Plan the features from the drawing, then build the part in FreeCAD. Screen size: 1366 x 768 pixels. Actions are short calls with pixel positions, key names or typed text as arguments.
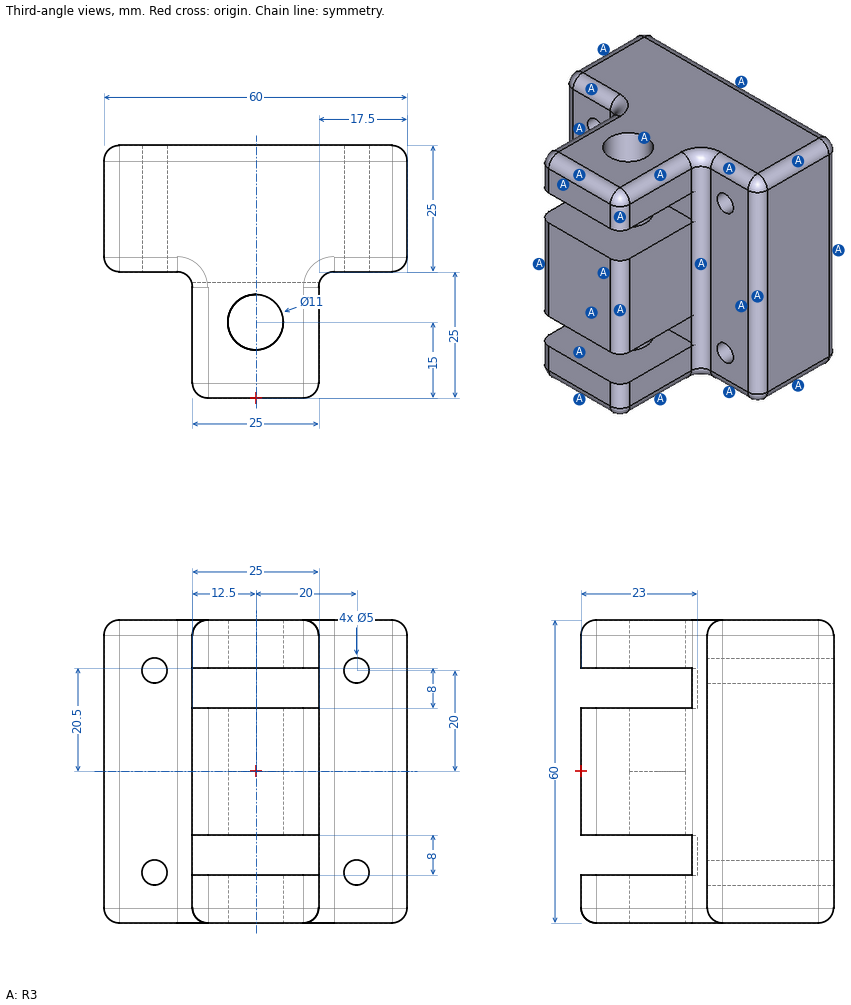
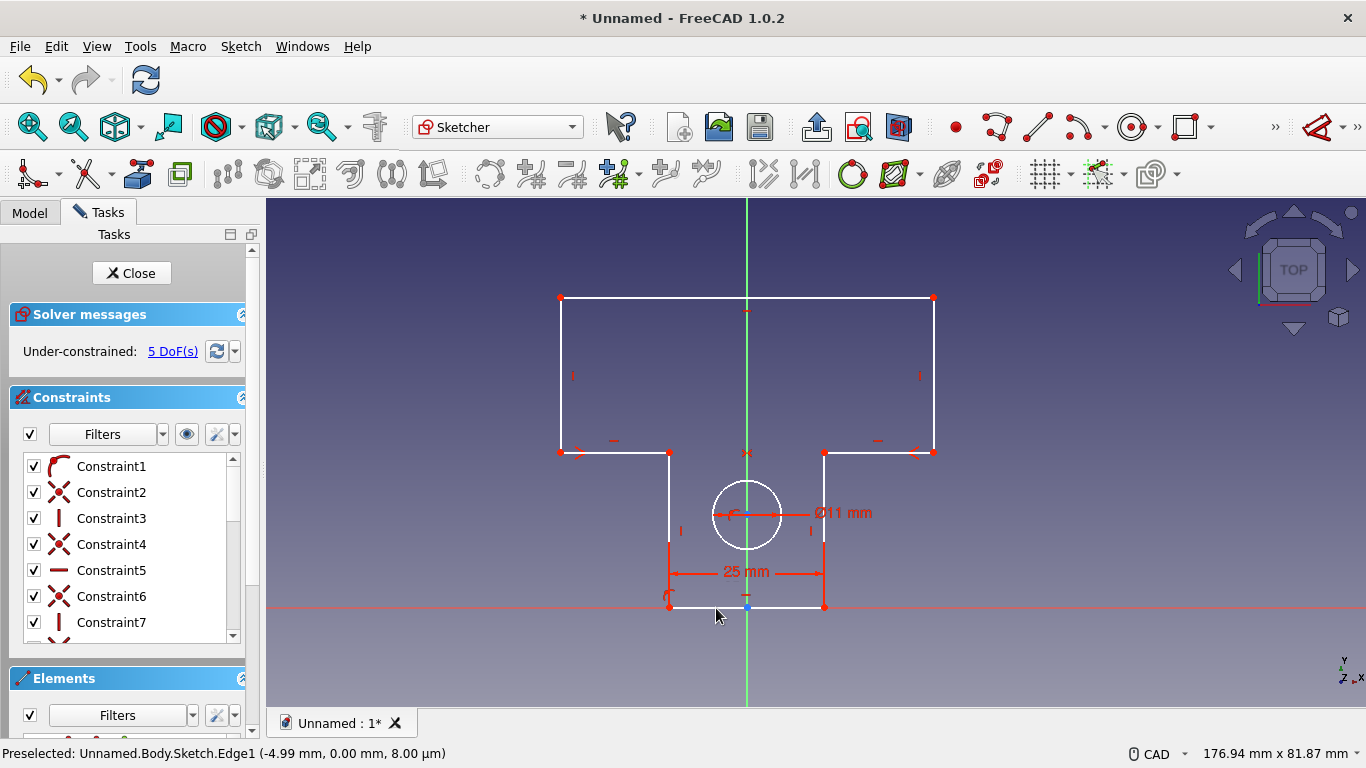
click(824, 561)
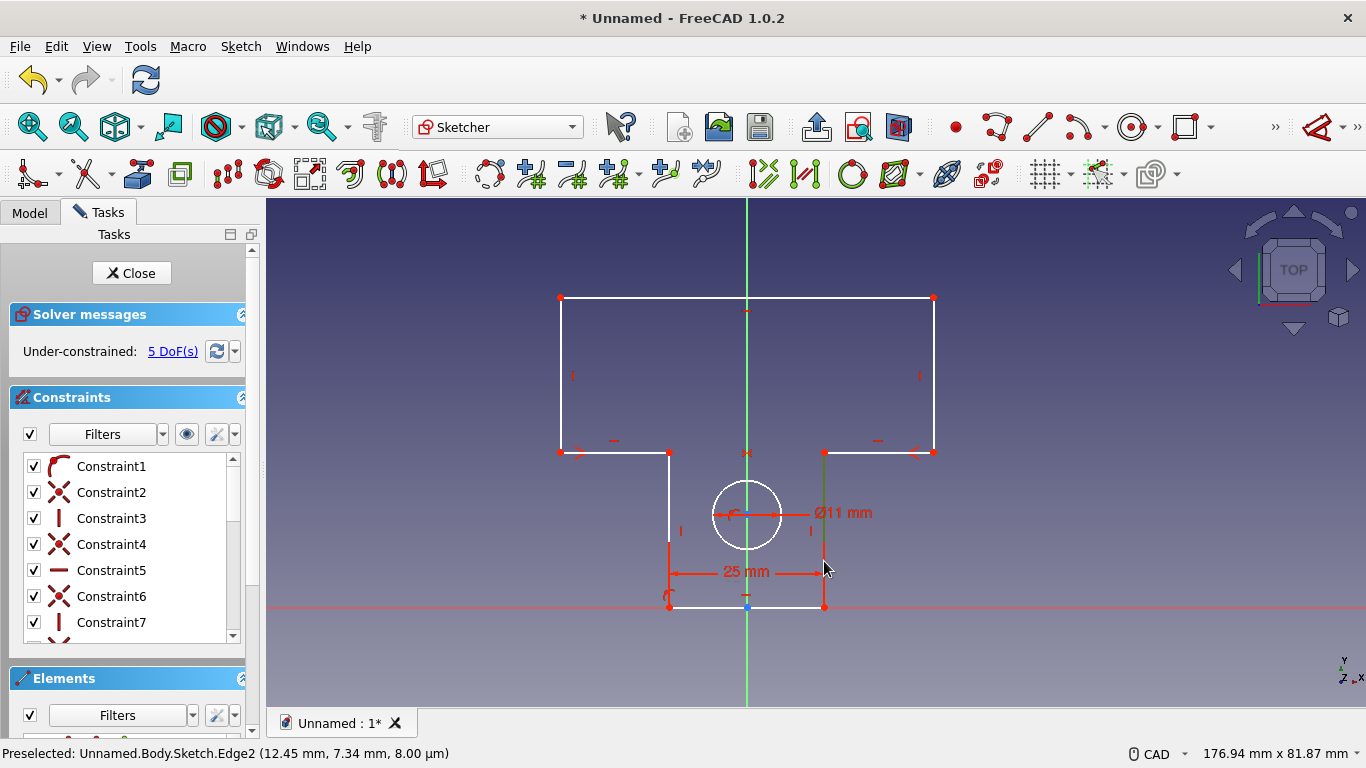
key(i)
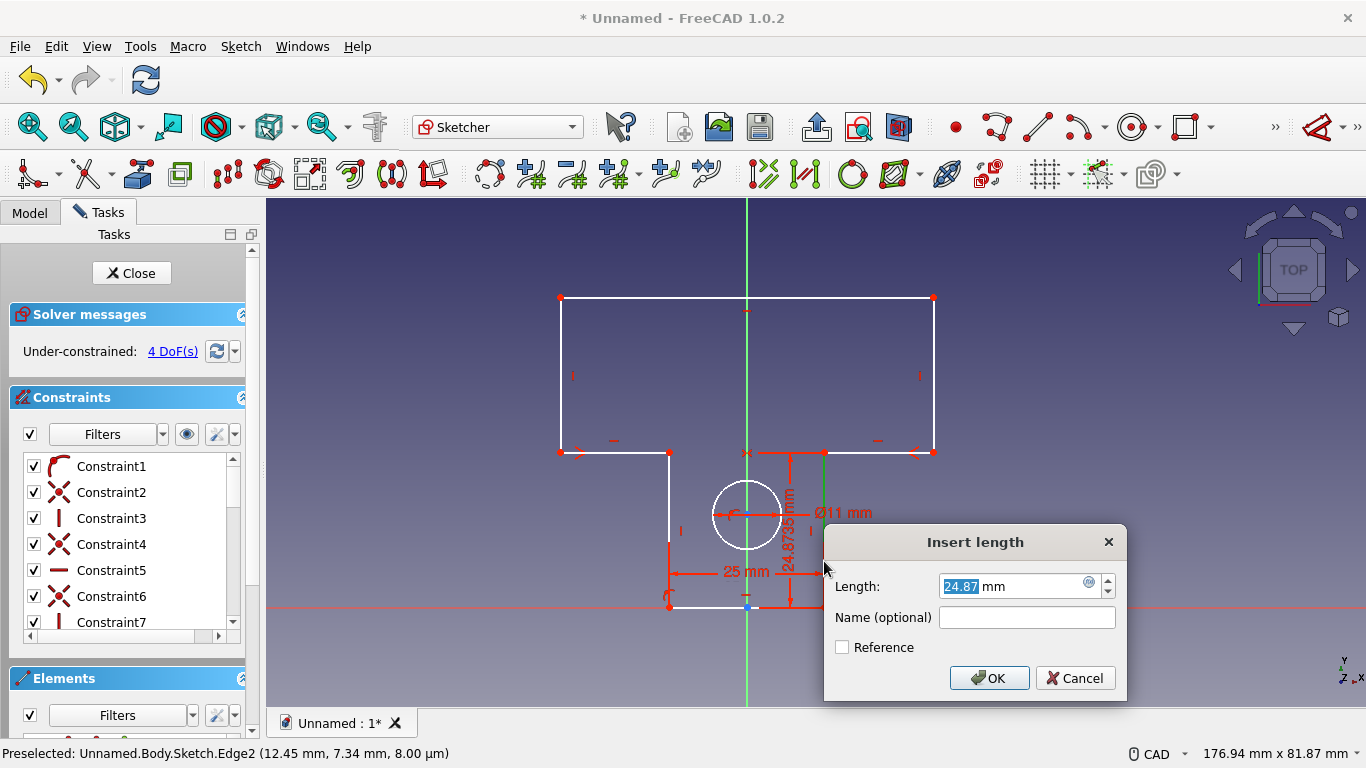
text(25)
key(Return)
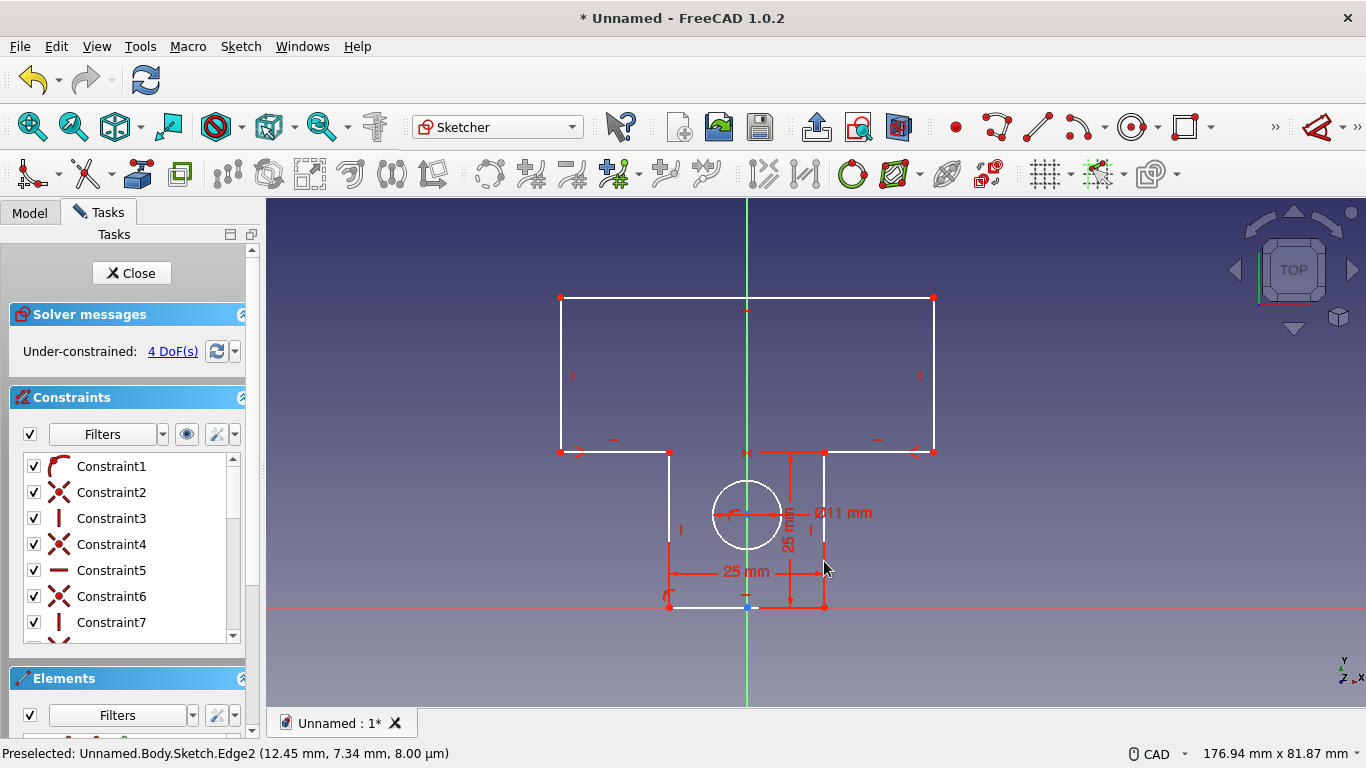
click(934, 406)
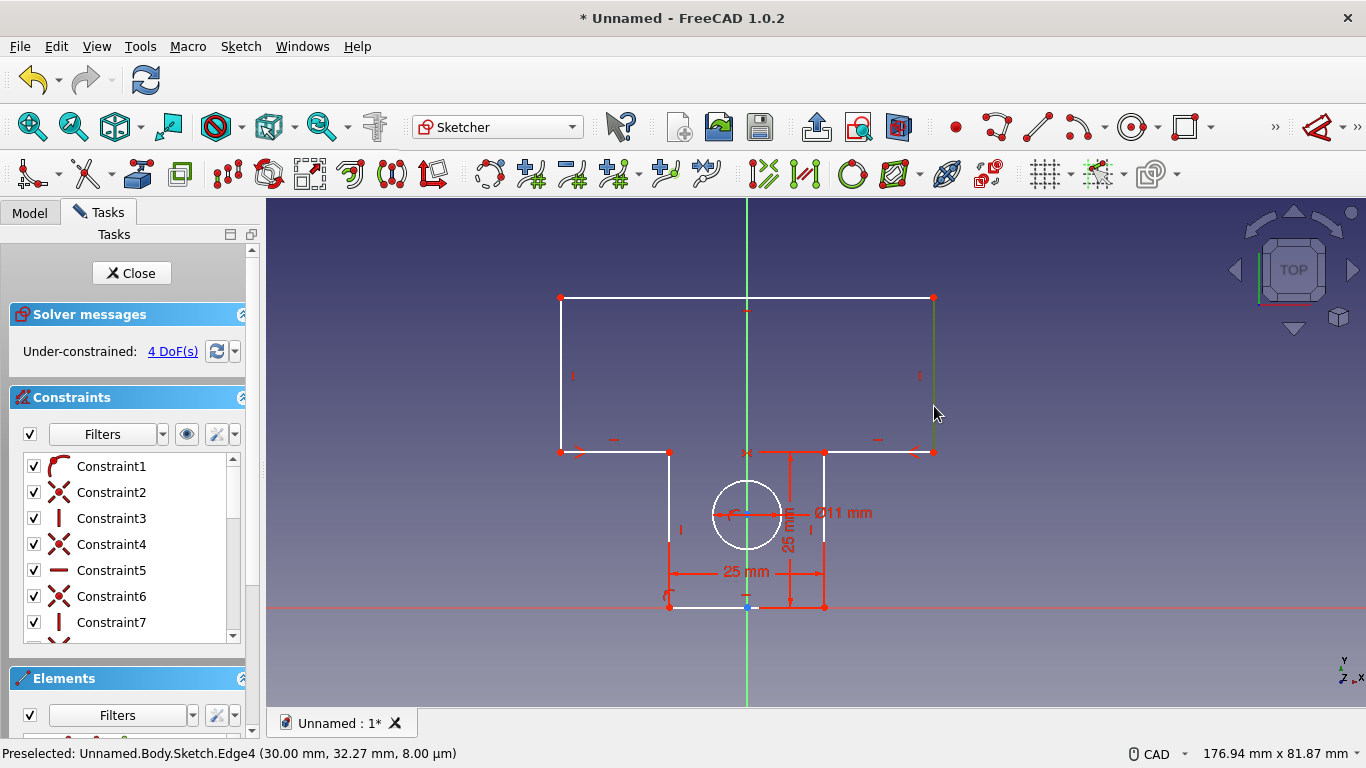
key(i)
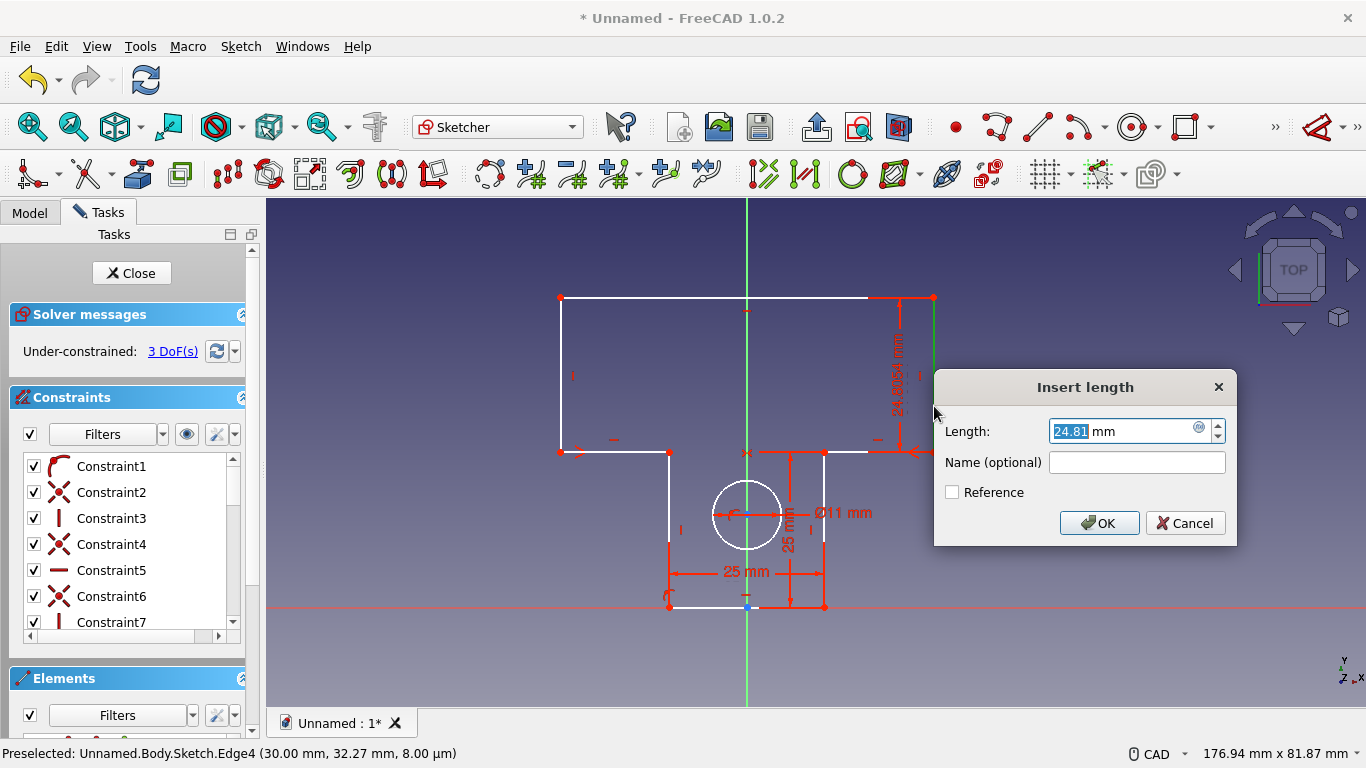
text(25)
key(Return)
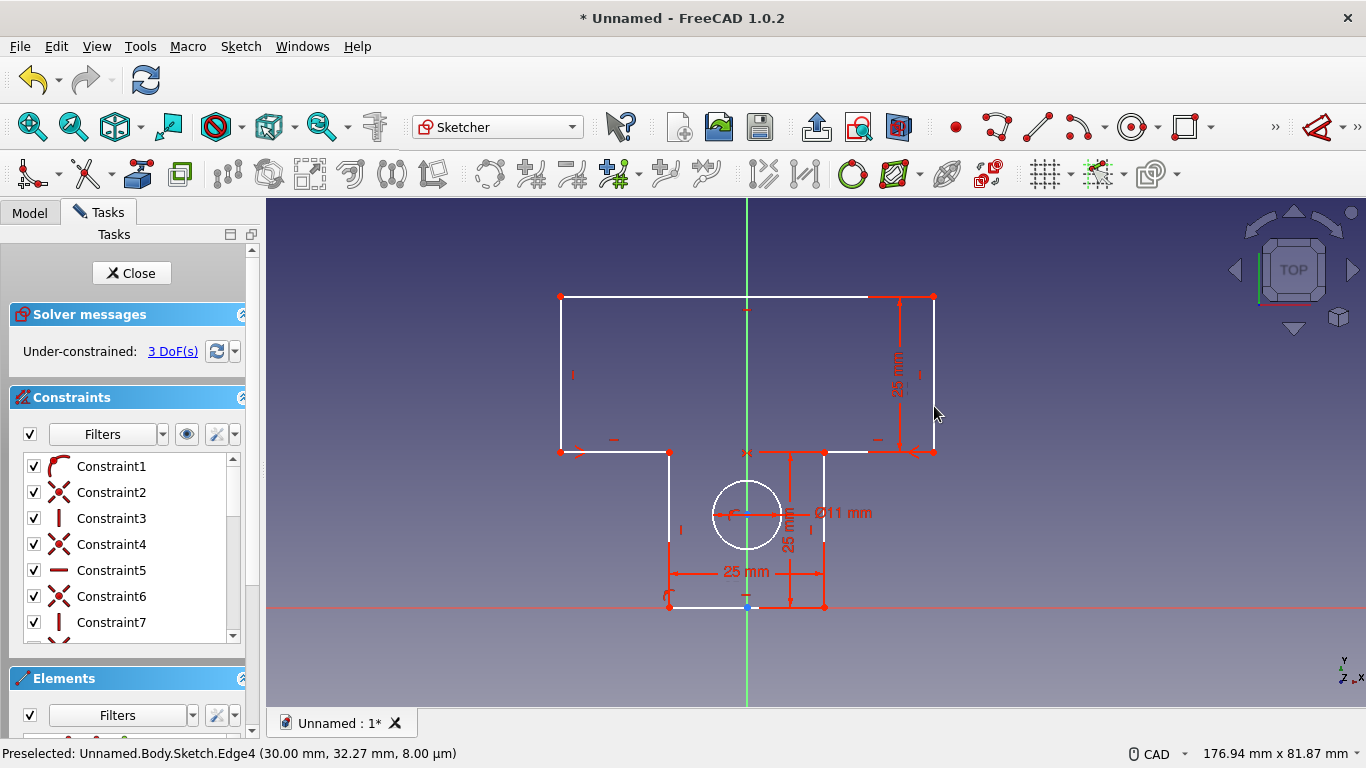
click(822, 297)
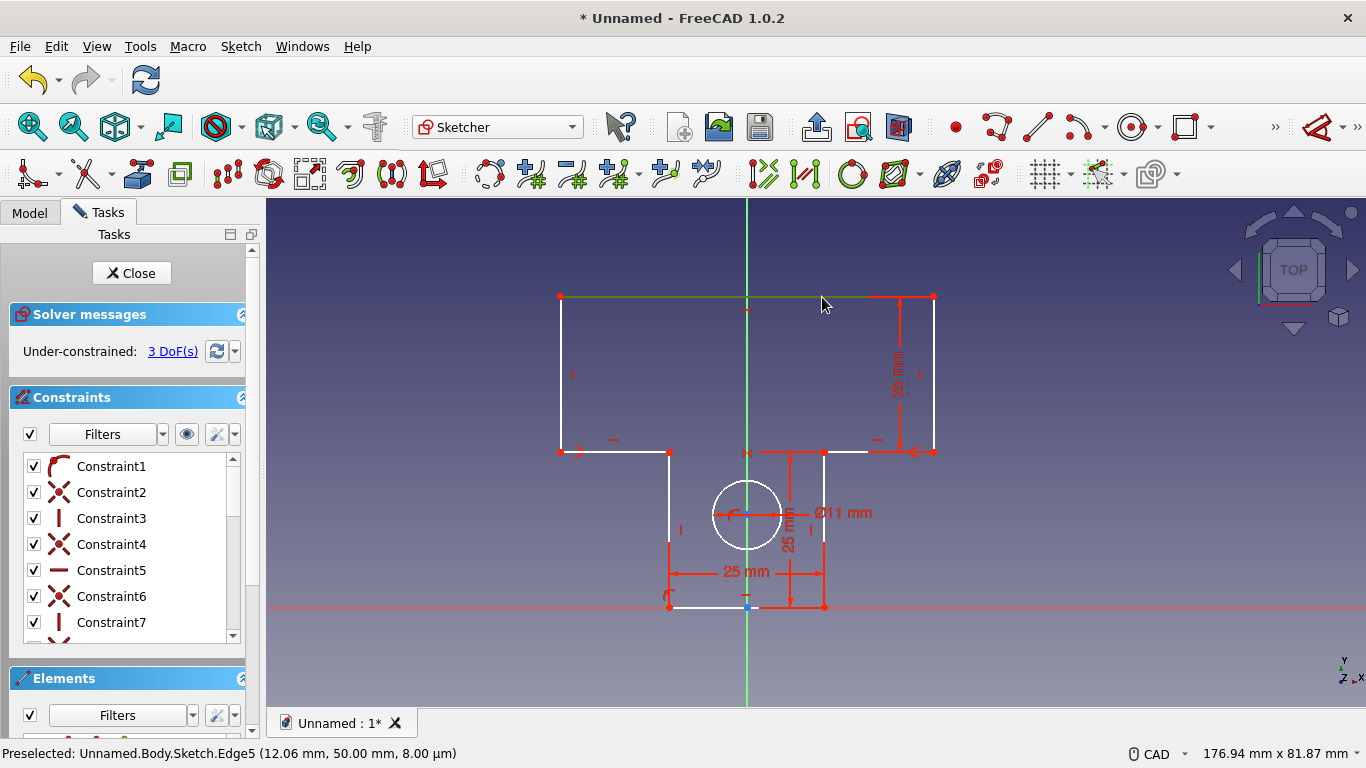
key(l)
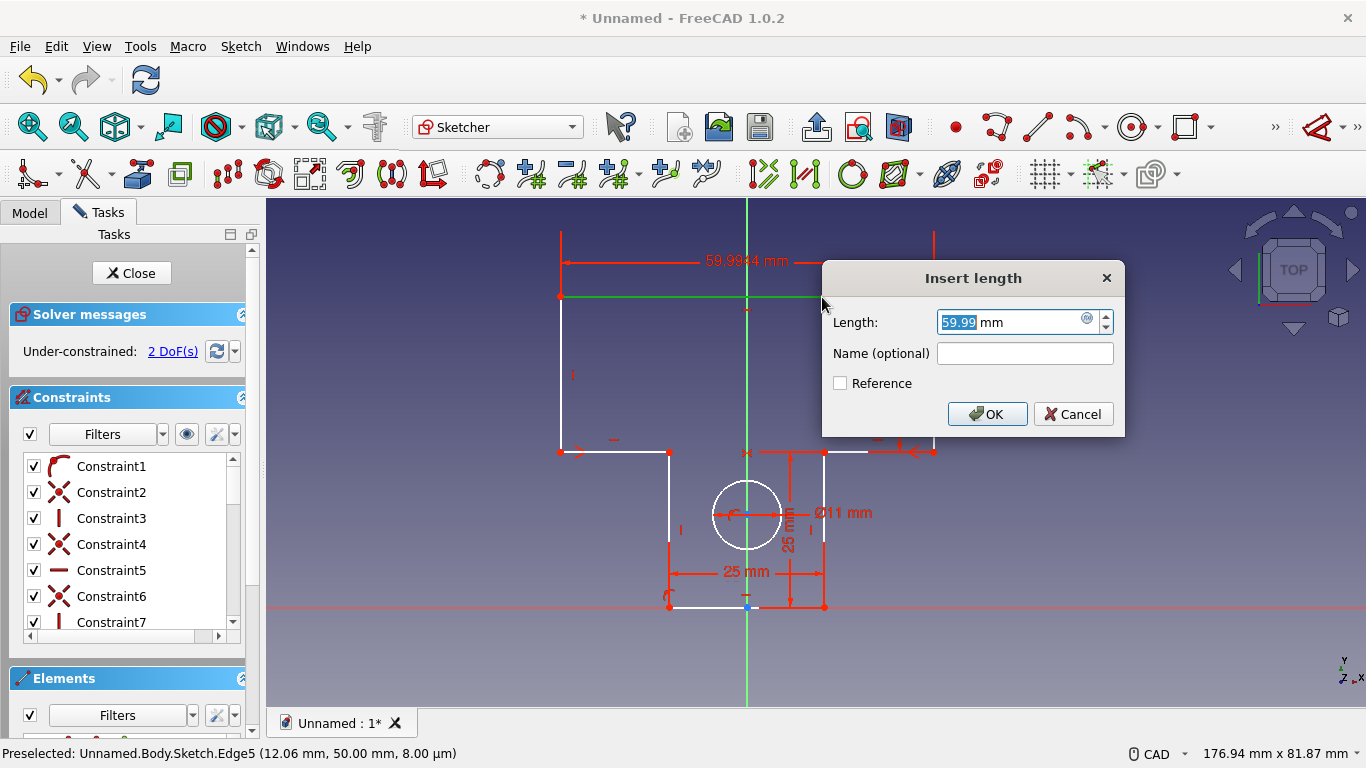
text(60)
key(Return)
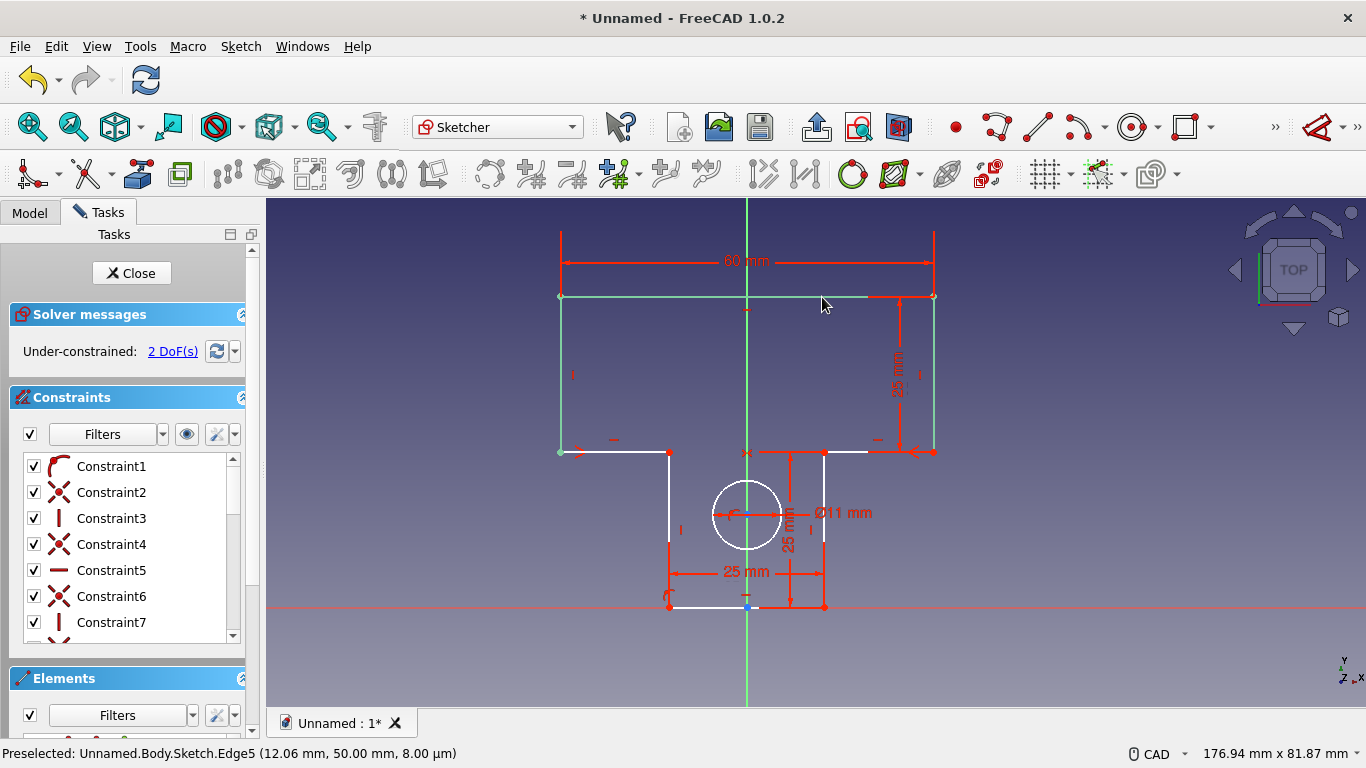
click(747, 515)